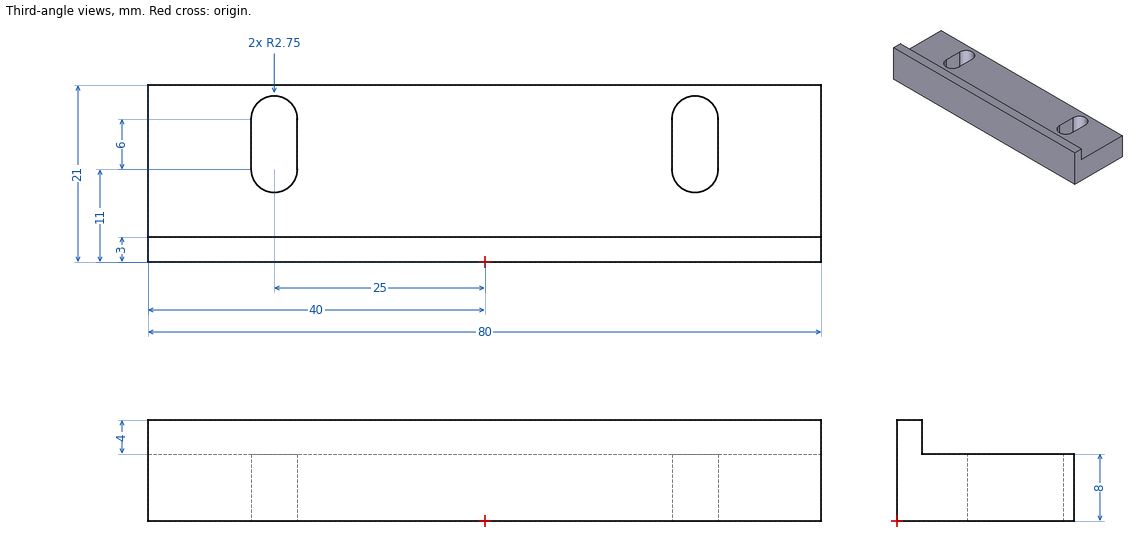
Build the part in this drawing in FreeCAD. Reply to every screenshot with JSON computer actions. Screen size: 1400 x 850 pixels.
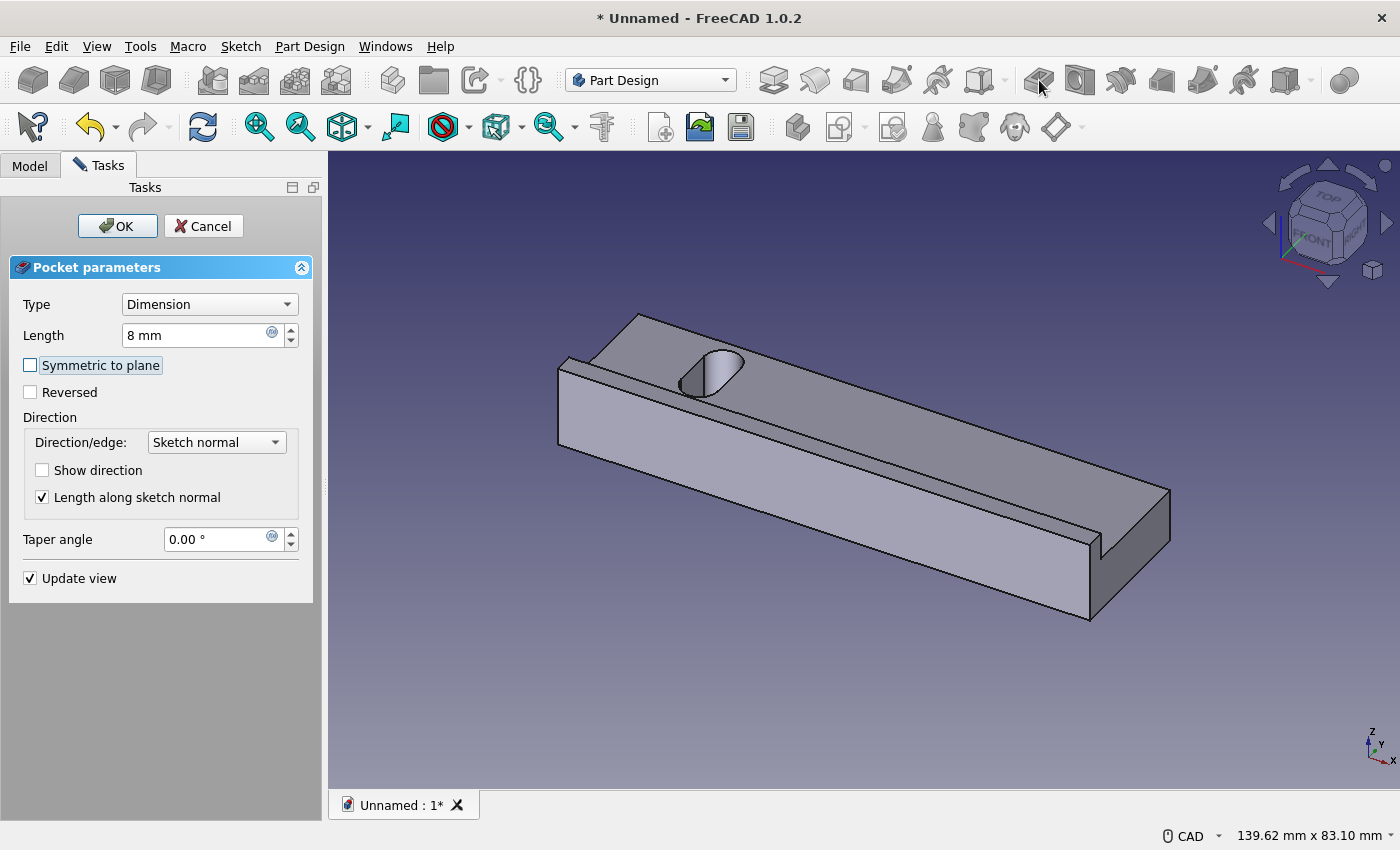
{"action": "left_click", "coordinate": [118, 226]}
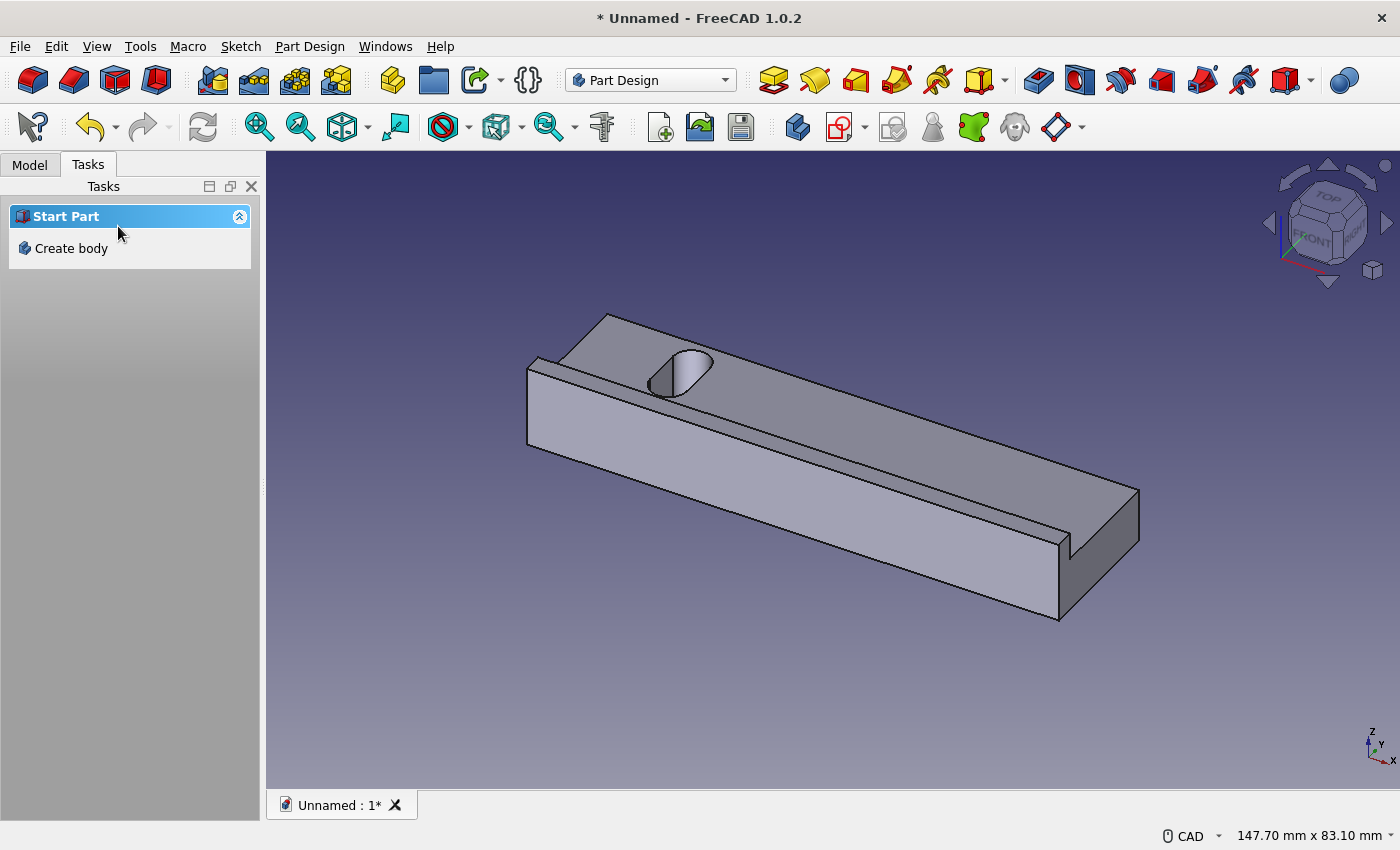
{"action": "left_click", "coordinate": [30, 164]}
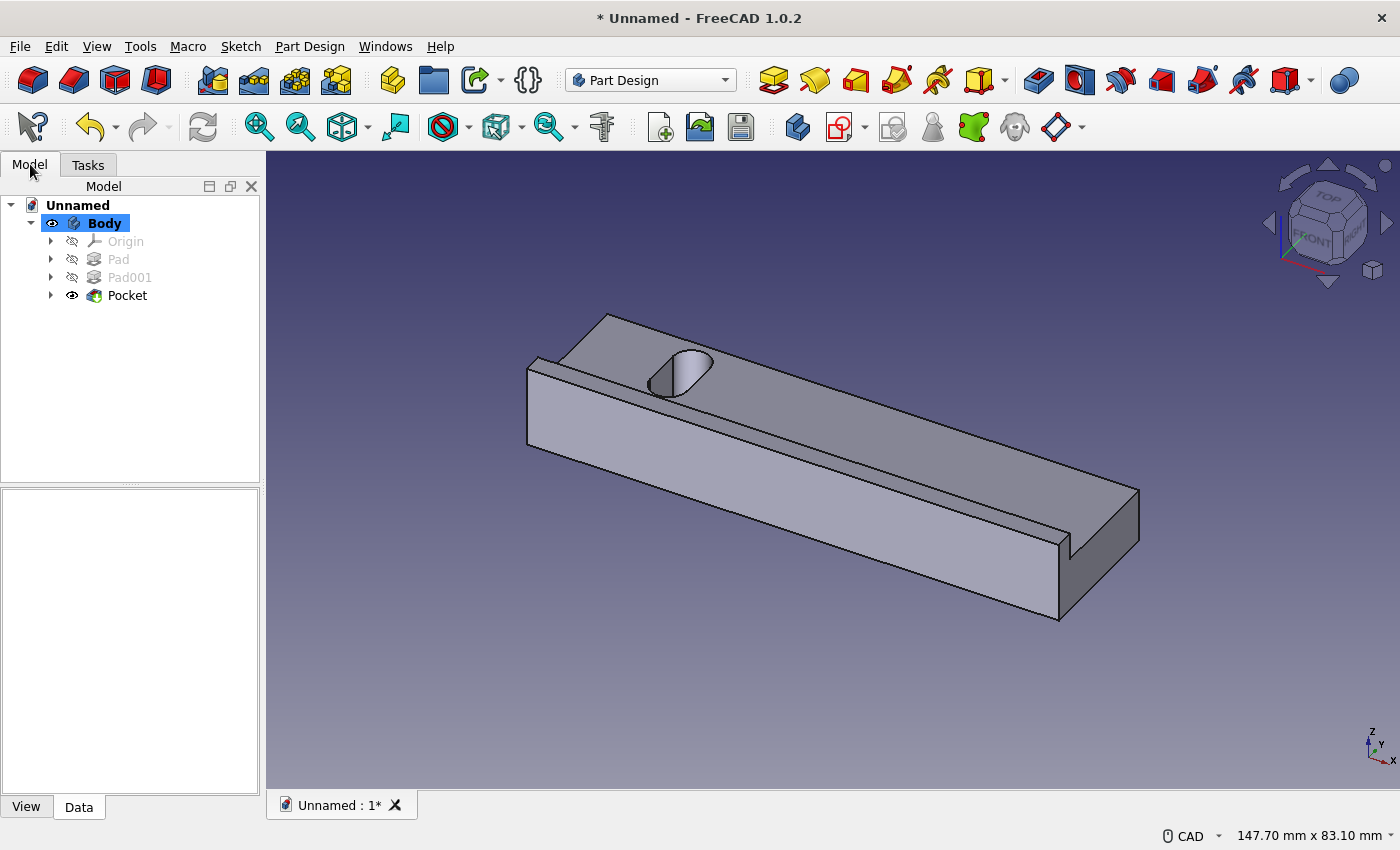
{"action": "left_click", "coordinate": [117, 295]}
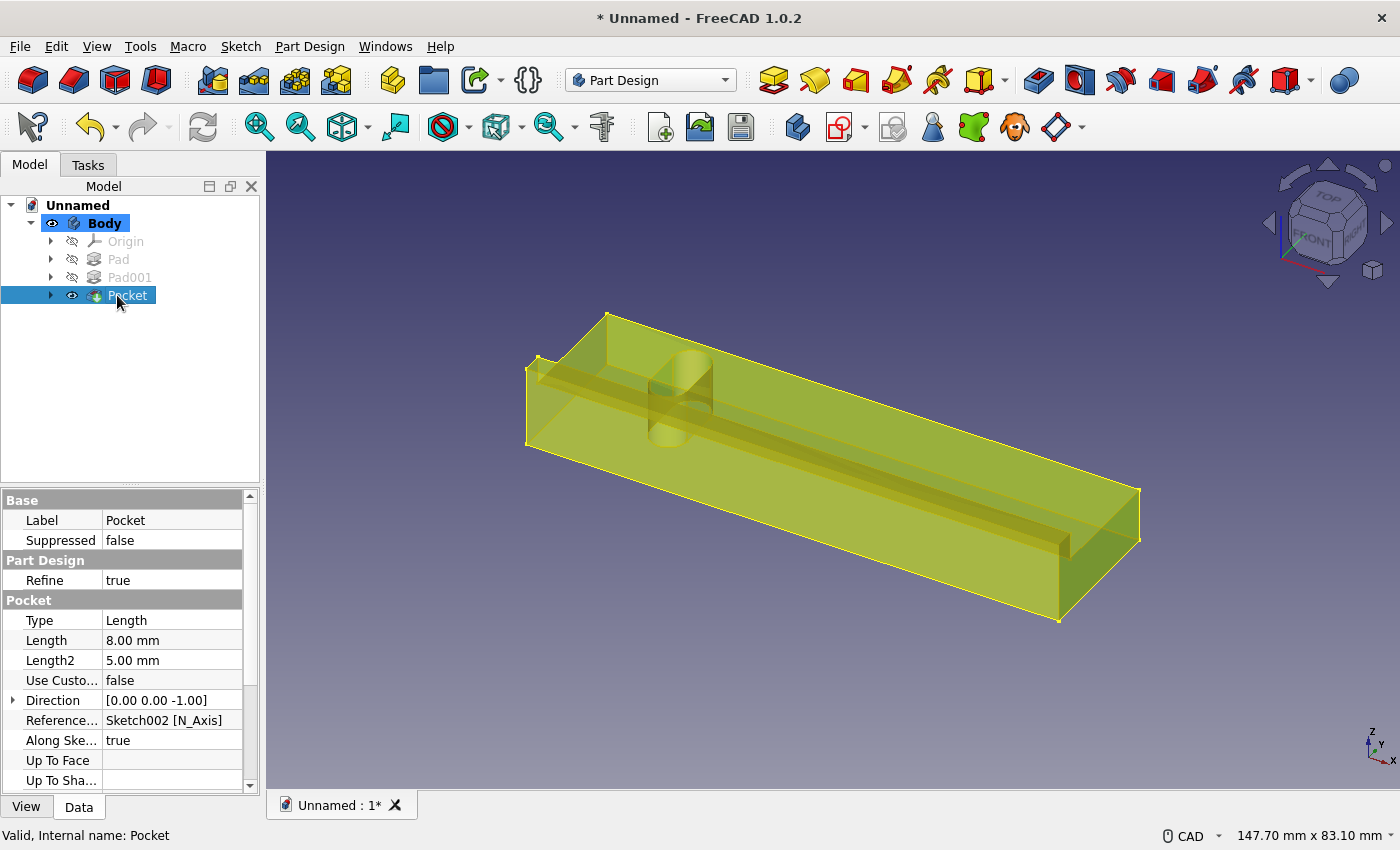
{"action": "left_click", "coordinate": [213, 80]}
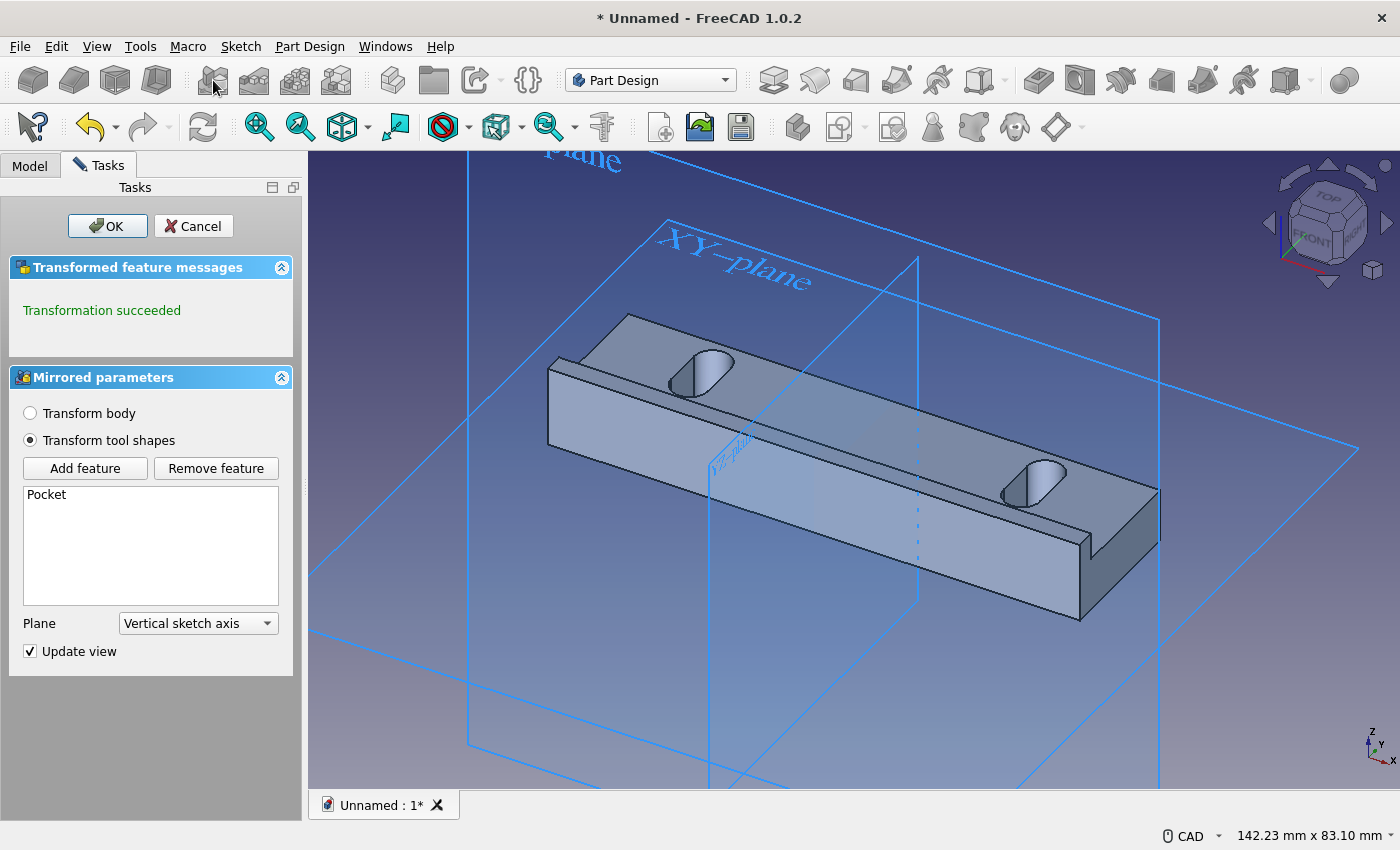
{"action": "left_click", "coordinate": [199, 624]}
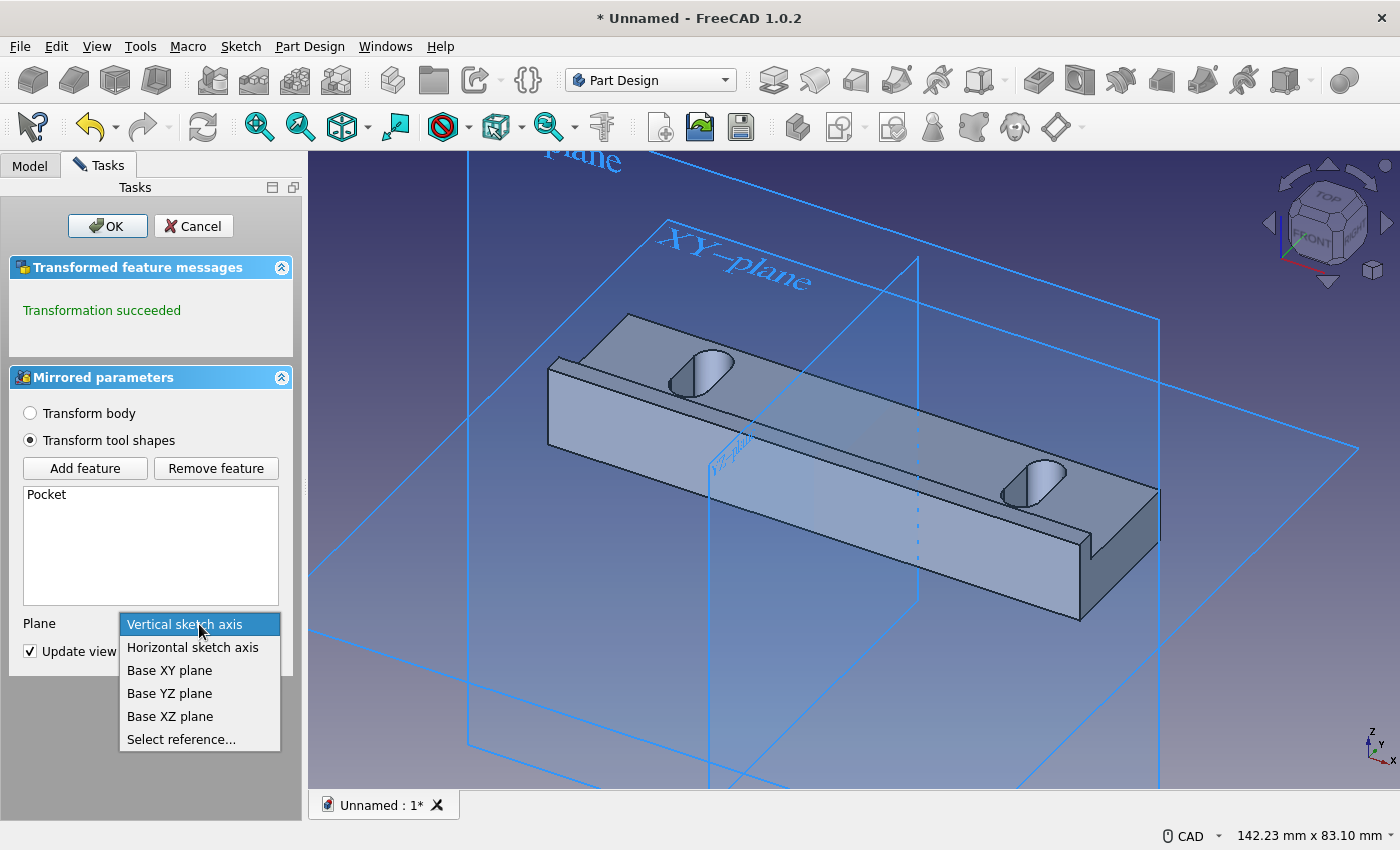
{"action": "left_click", "coordinate": [198, 694]}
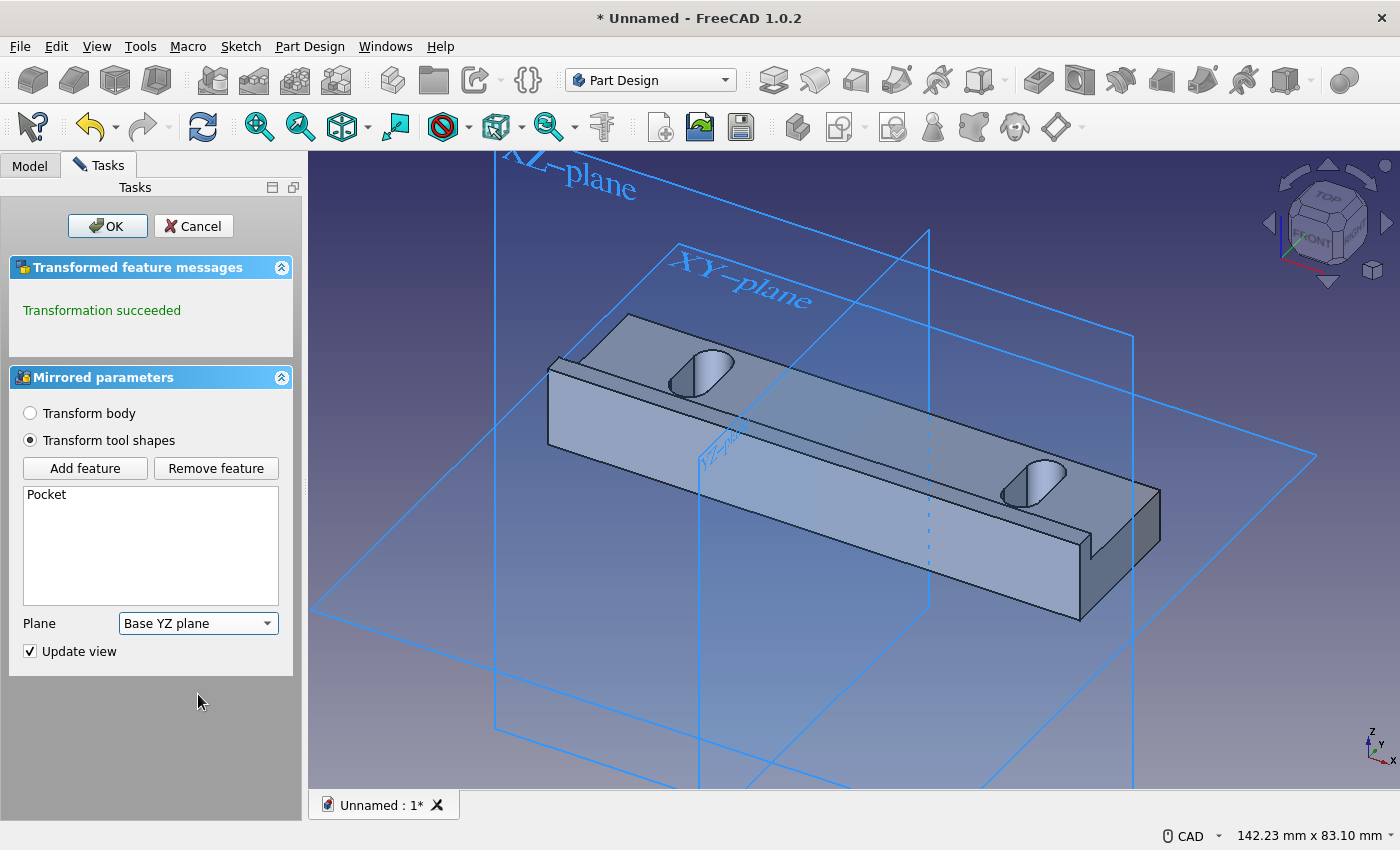
{"action": "left_click", "coordinate": [108, 226]}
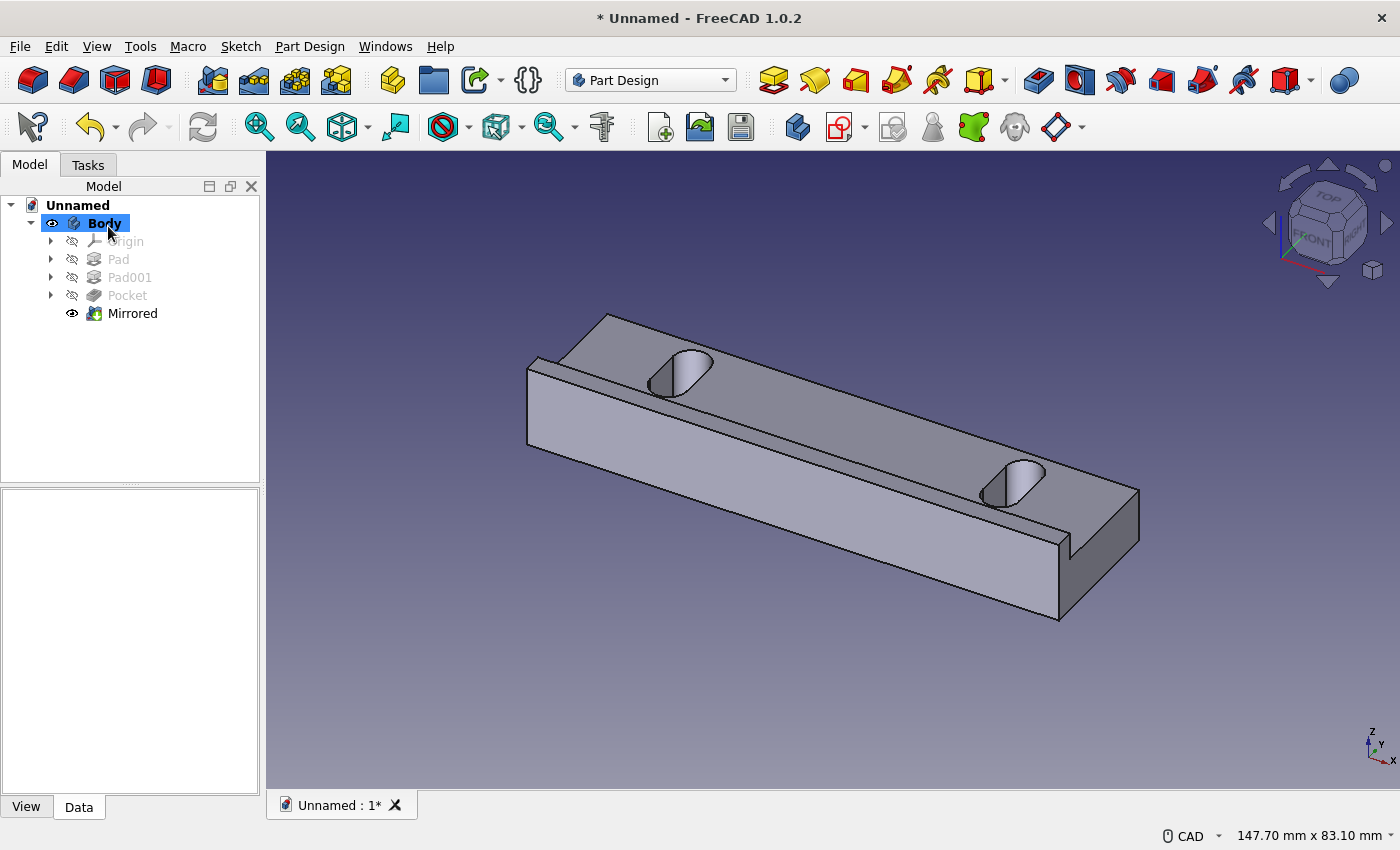
{"action": "key", "text": "0"}